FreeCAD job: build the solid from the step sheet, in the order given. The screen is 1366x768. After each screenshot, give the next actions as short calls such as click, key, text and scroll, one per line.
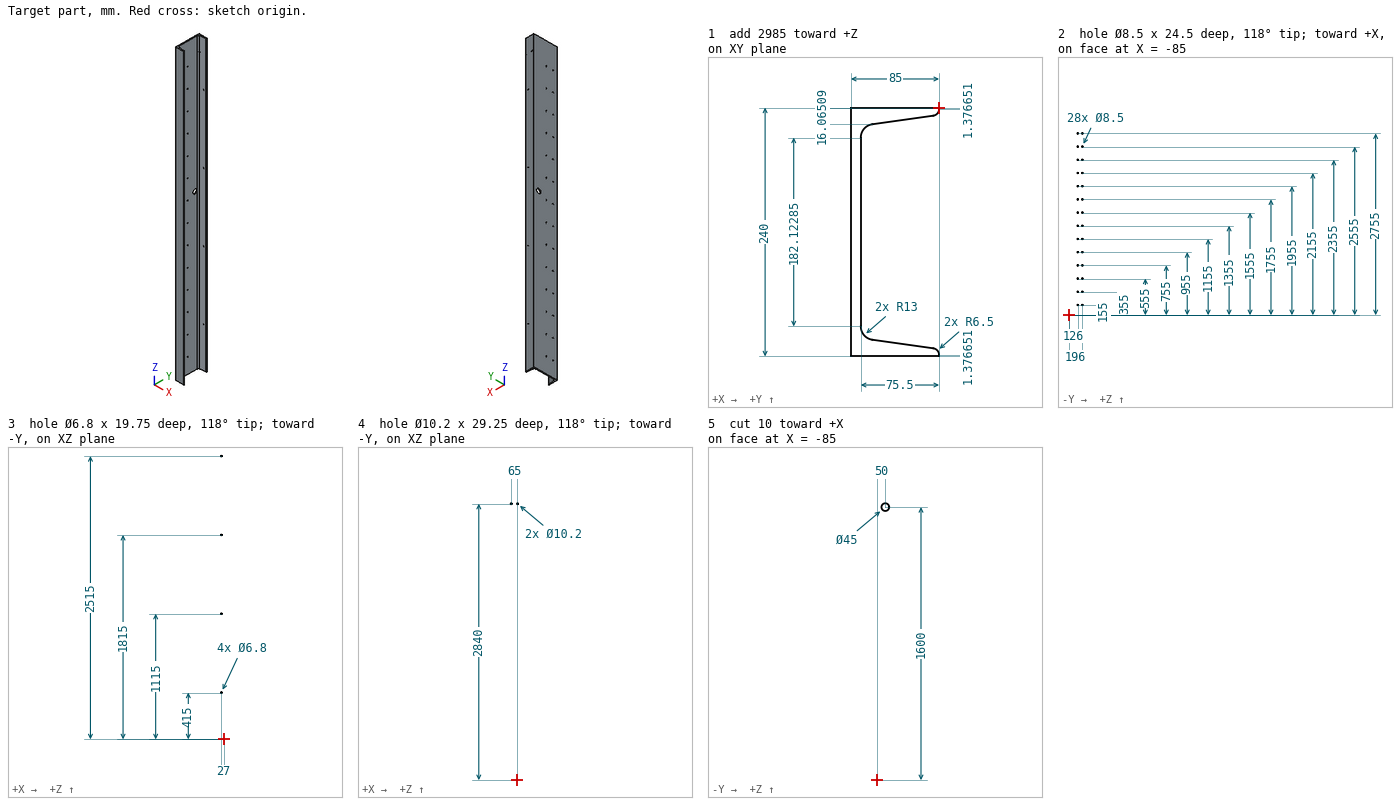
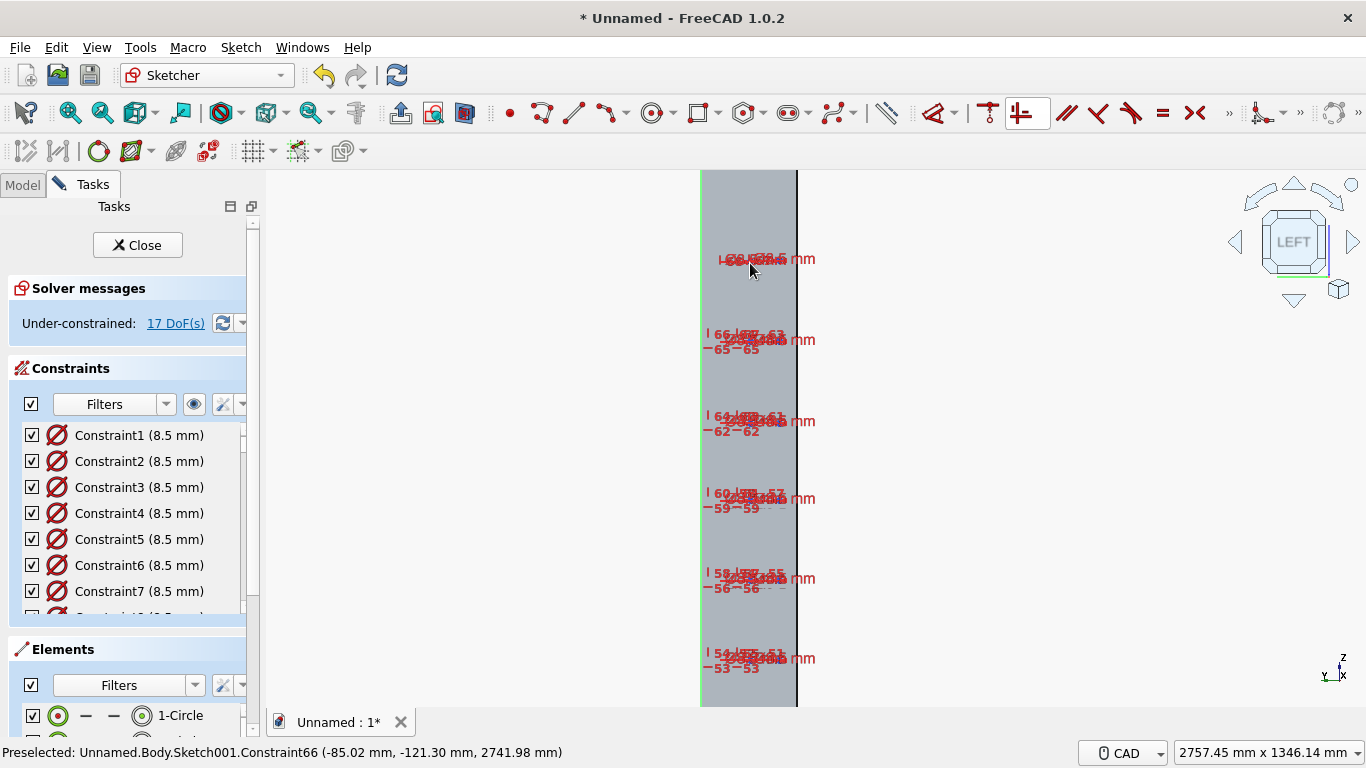
scroll(750, 262, up, 4)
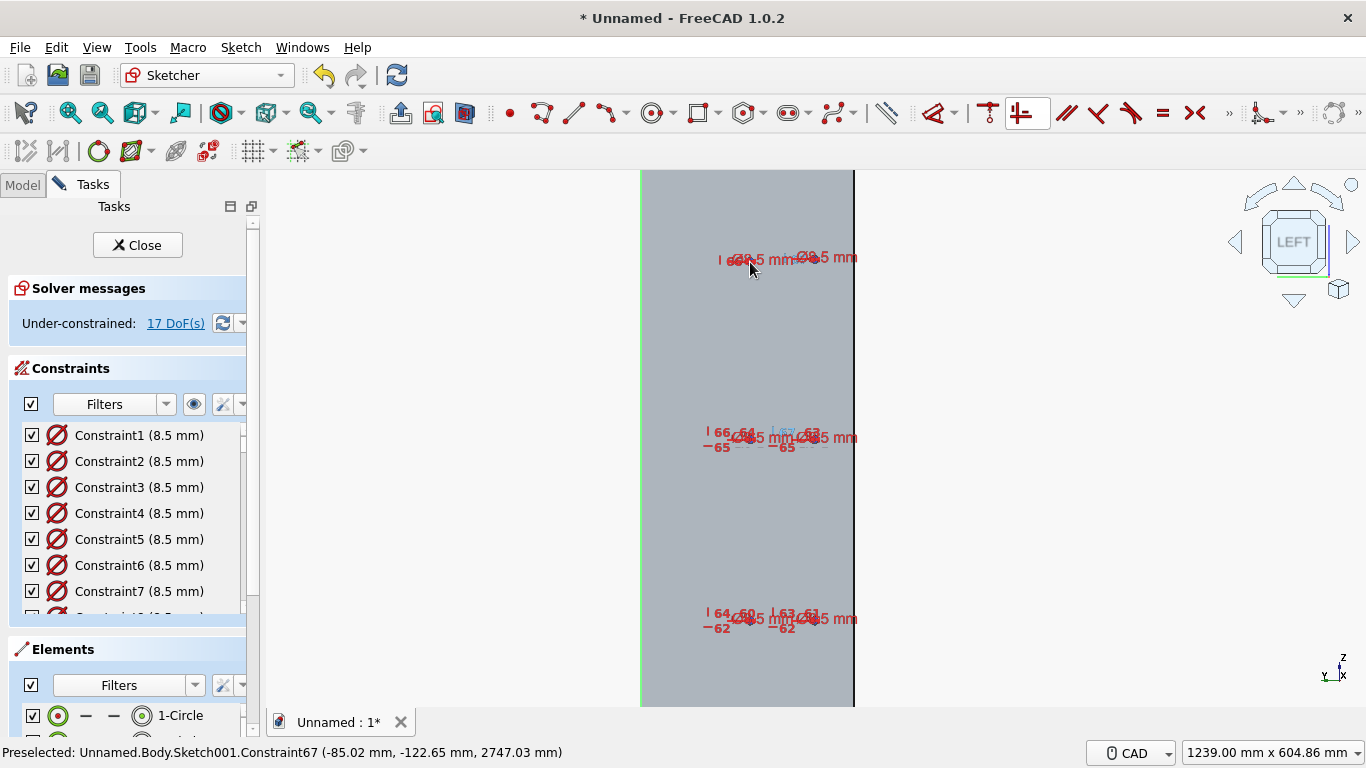
click(750, 262)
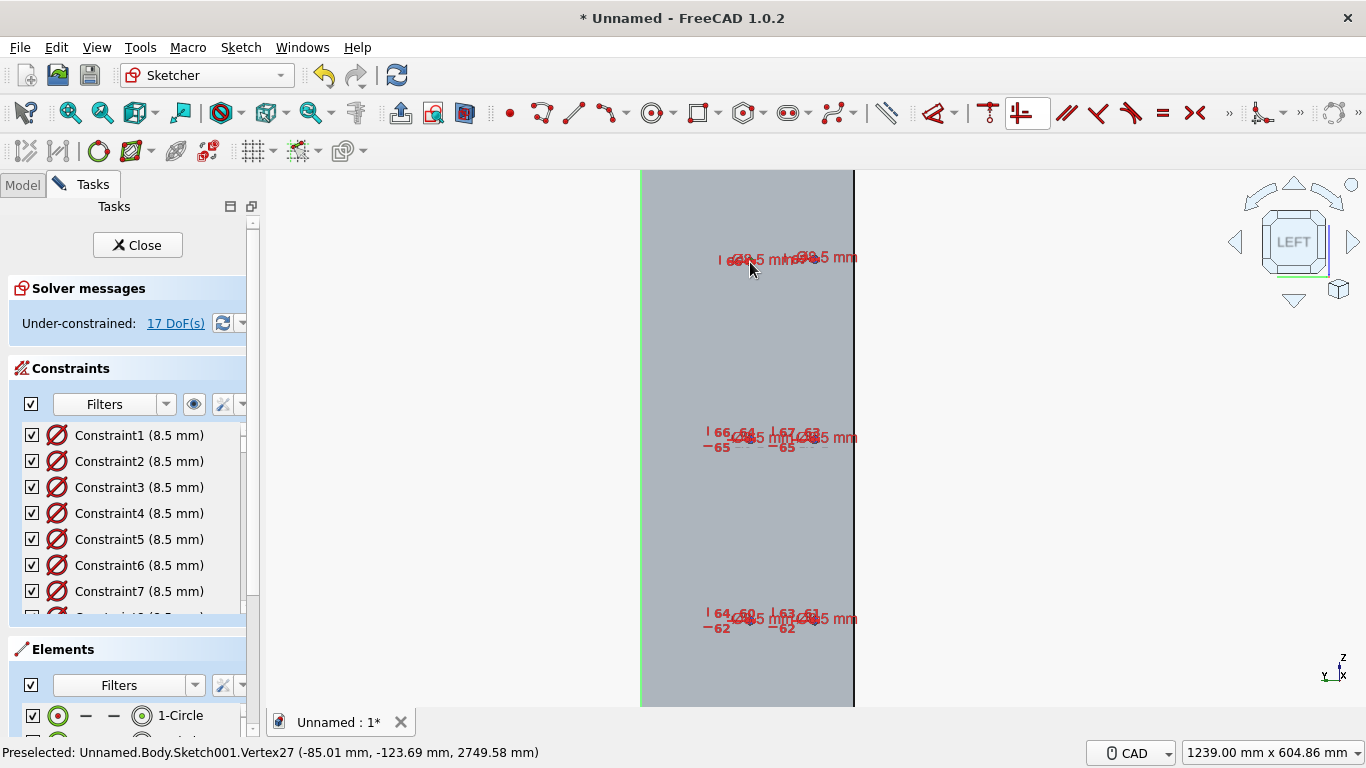
scroll(750, 276, down, 10)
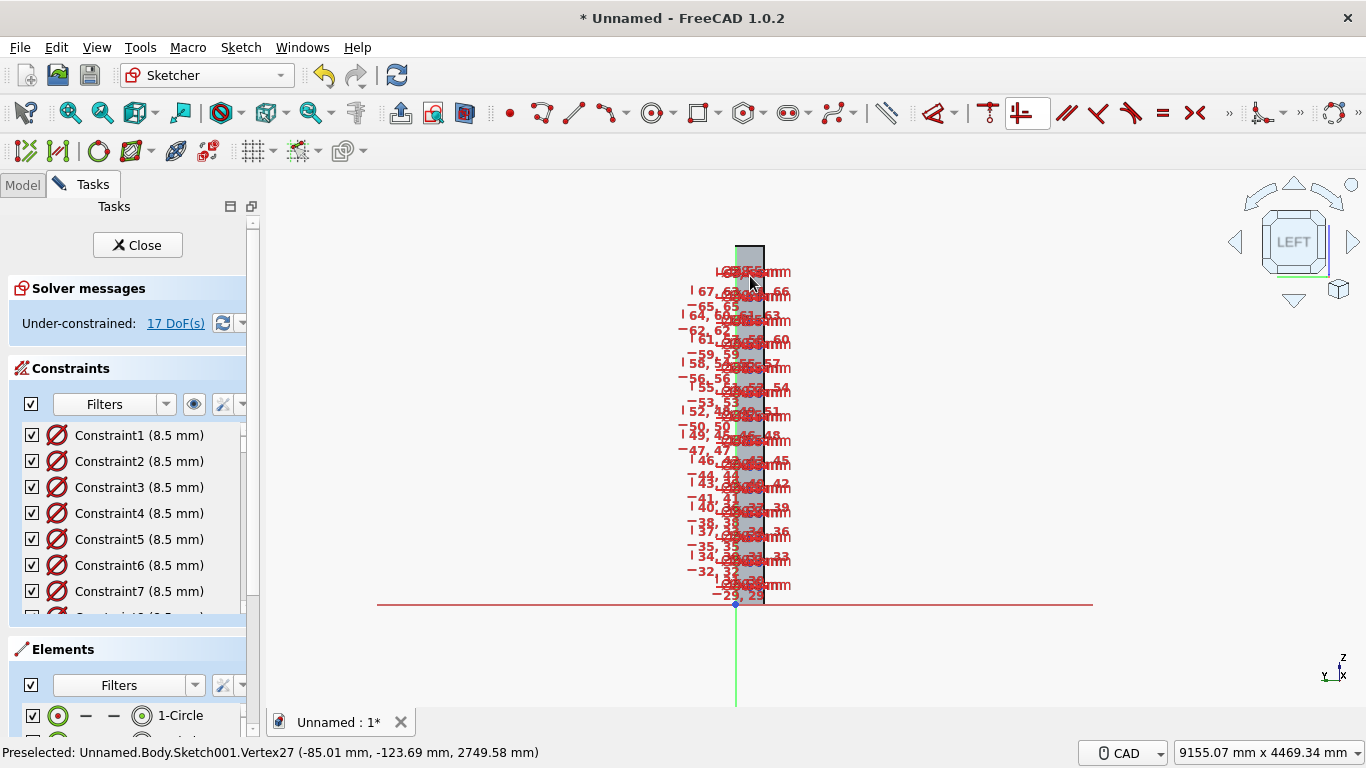
scroll(759, 274, up, 2)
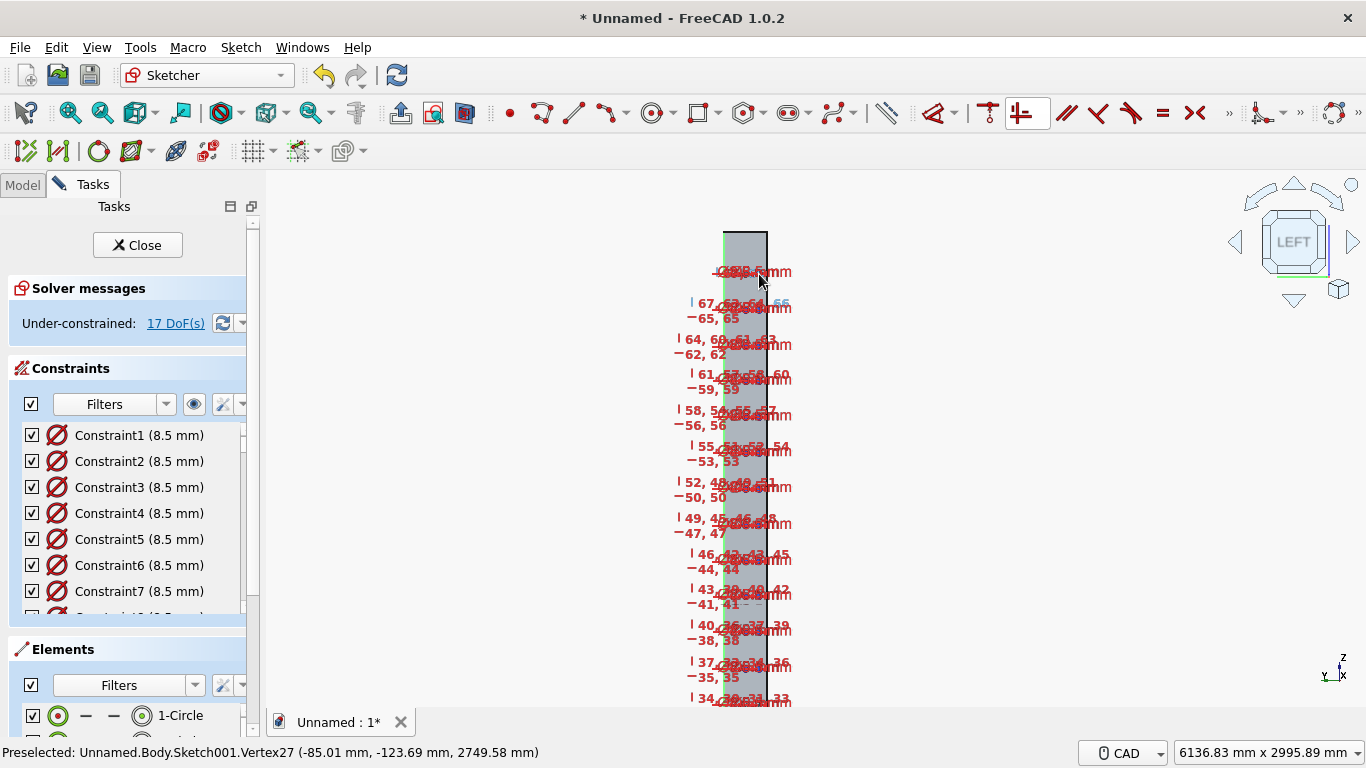
scroll(759, 274, up, 4)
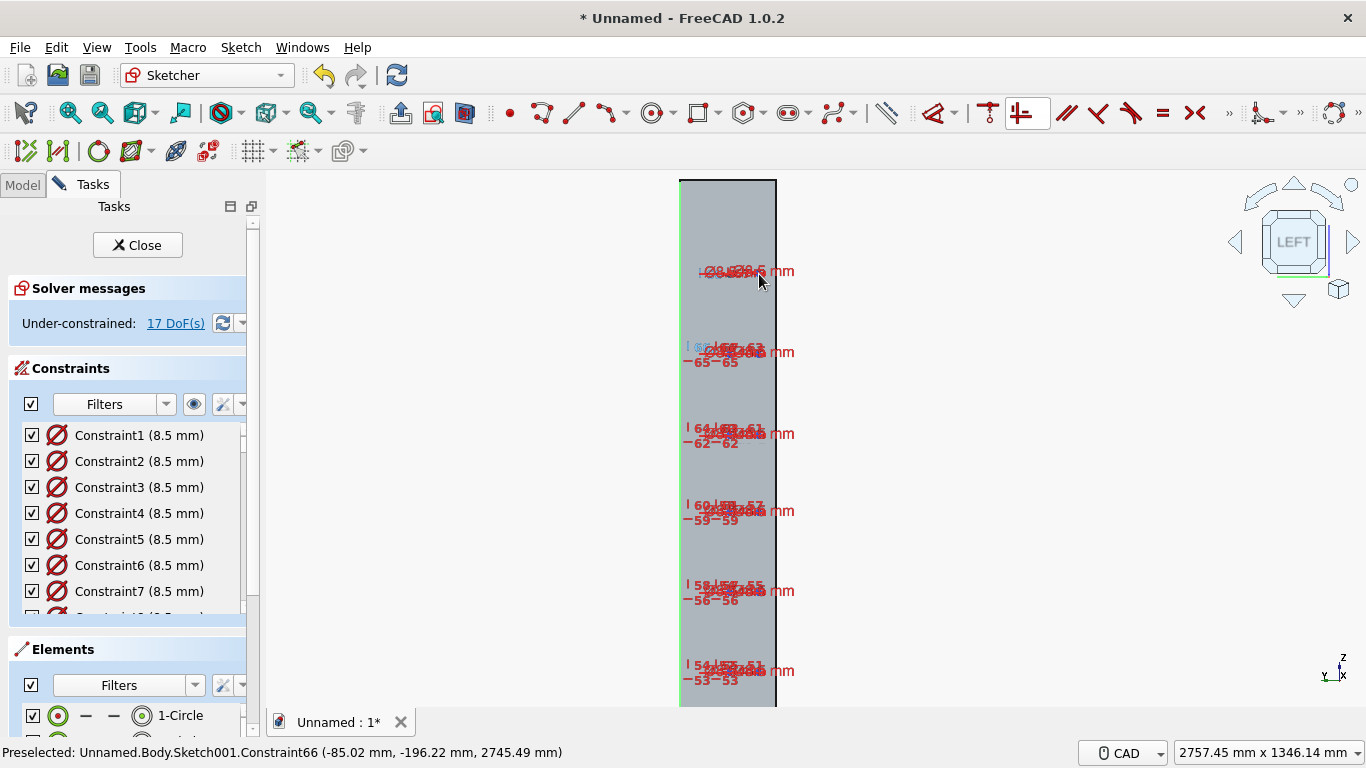
click(758, 273)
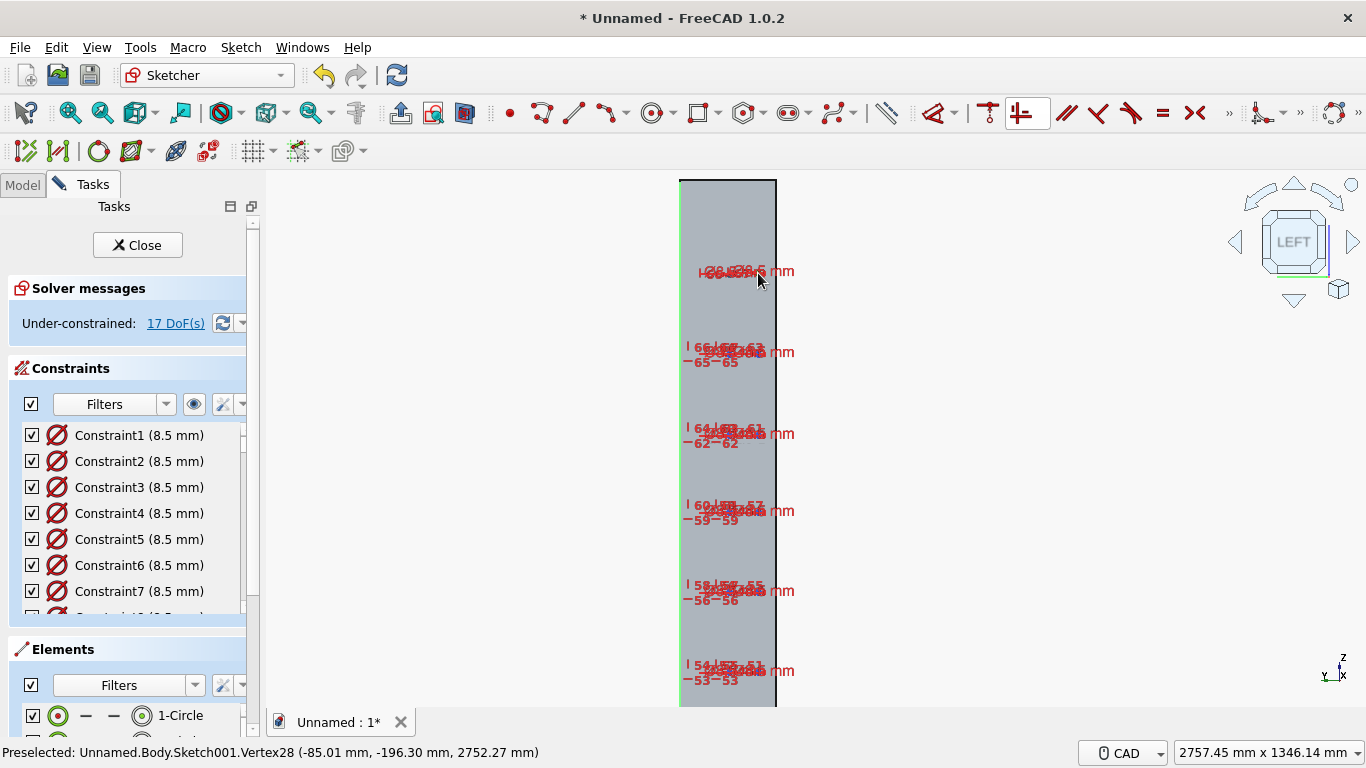
click(1044, 114)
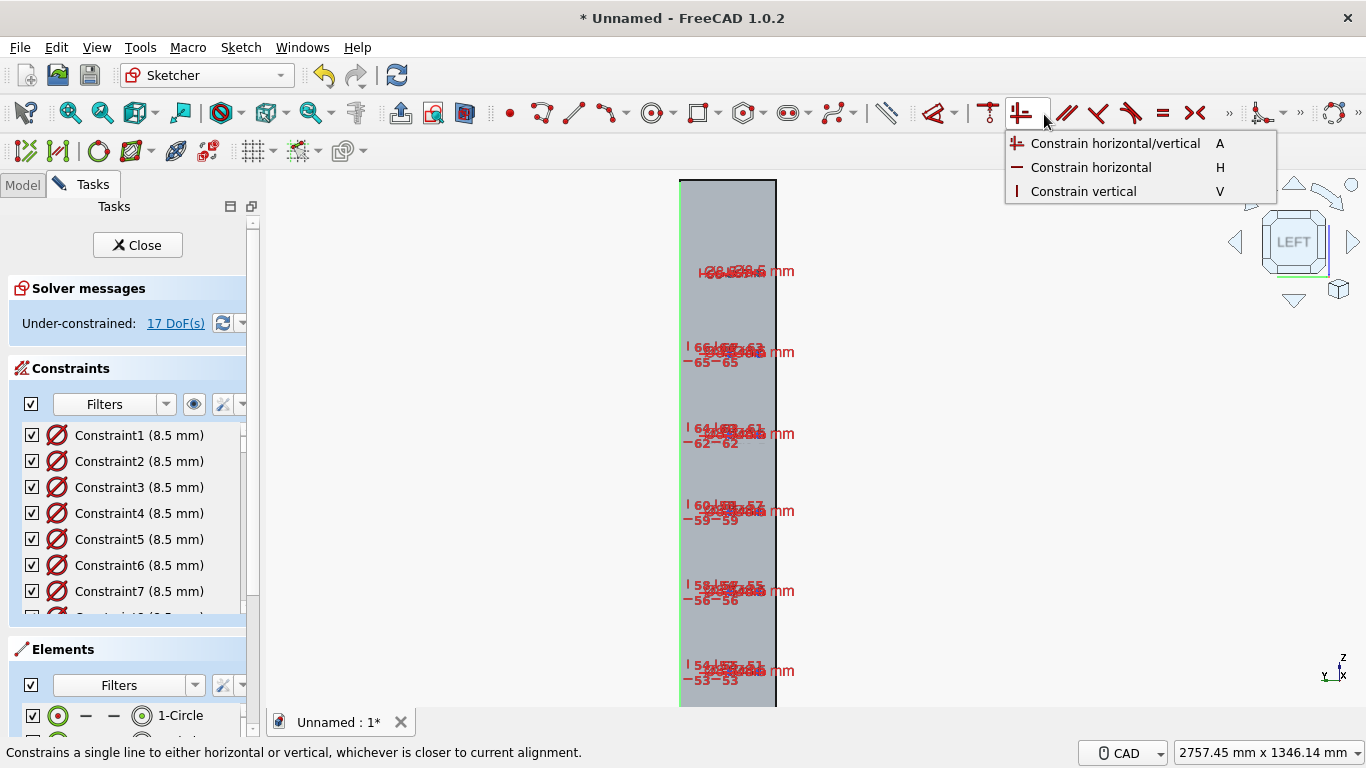
click(1141, 167)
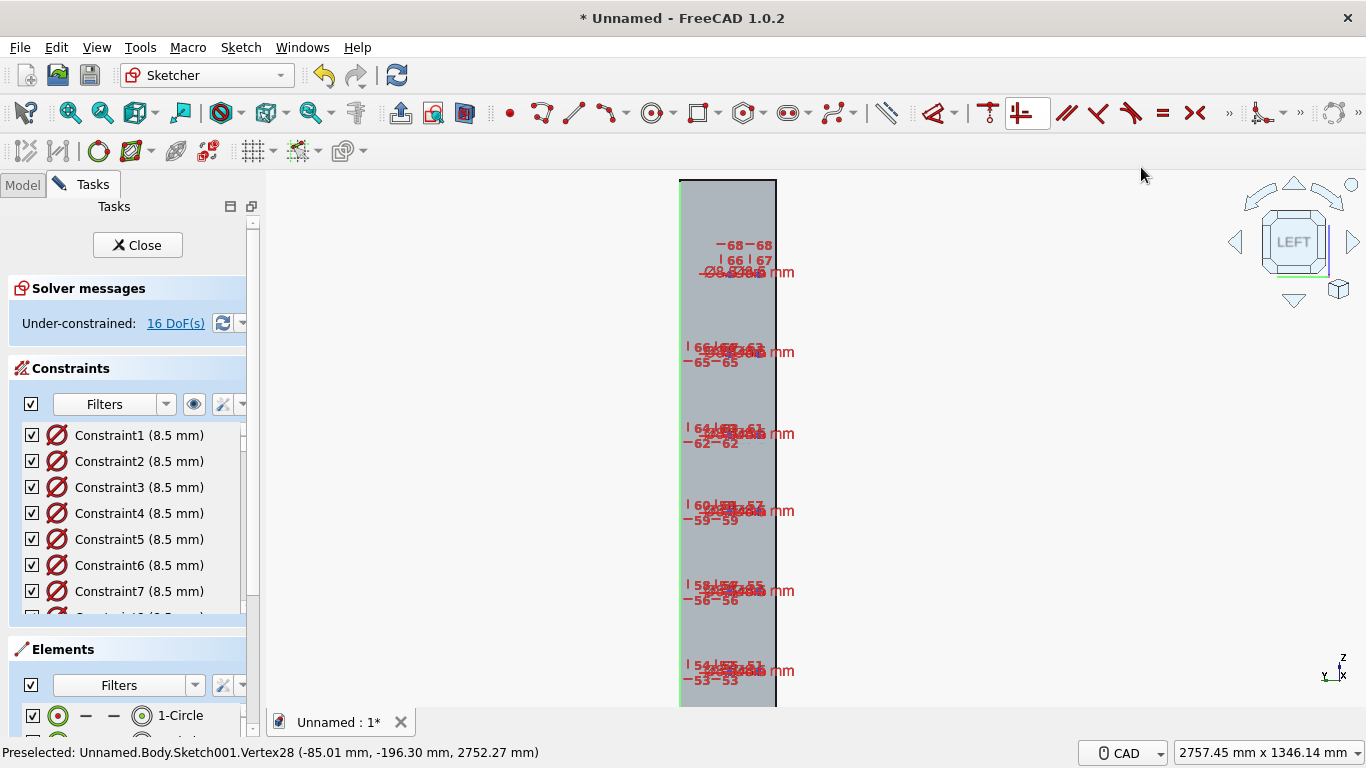
click(934, 114)